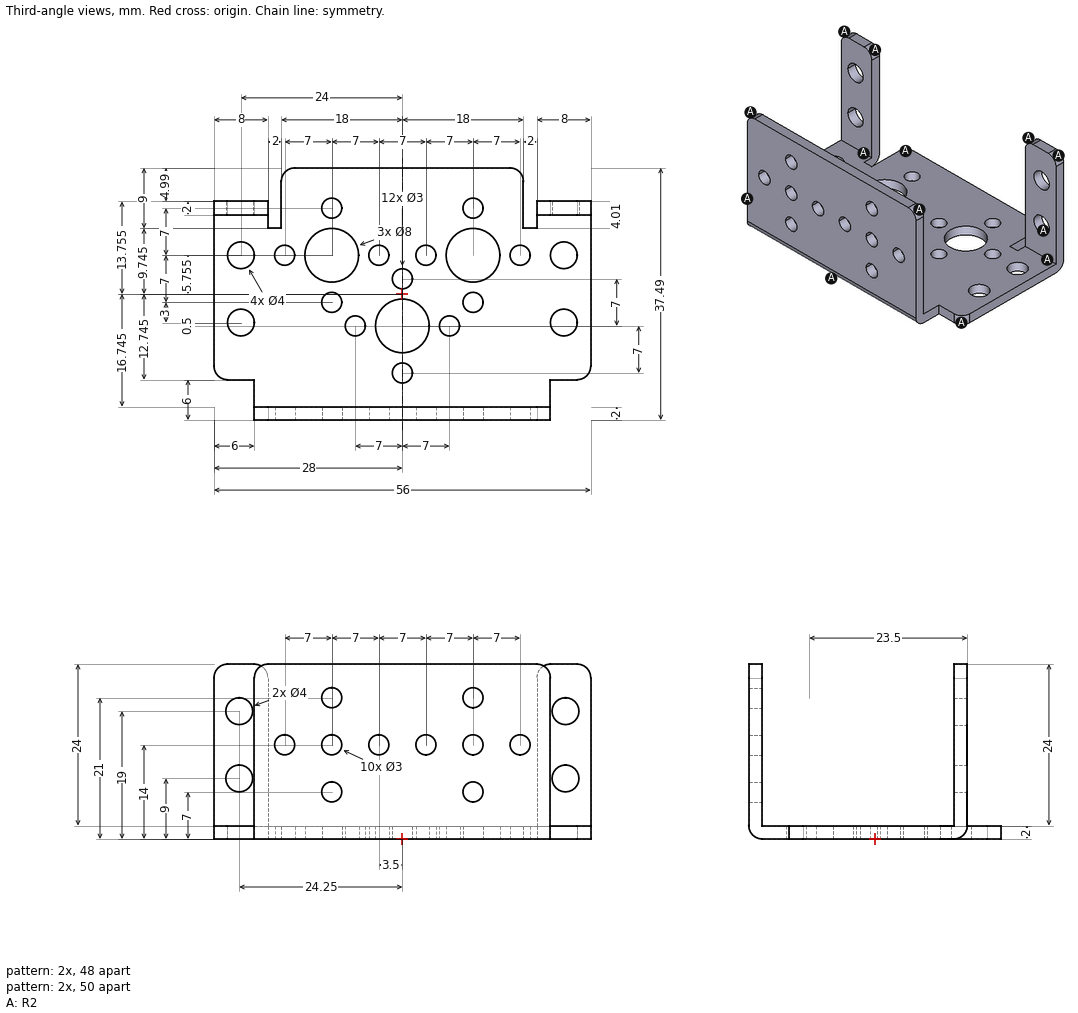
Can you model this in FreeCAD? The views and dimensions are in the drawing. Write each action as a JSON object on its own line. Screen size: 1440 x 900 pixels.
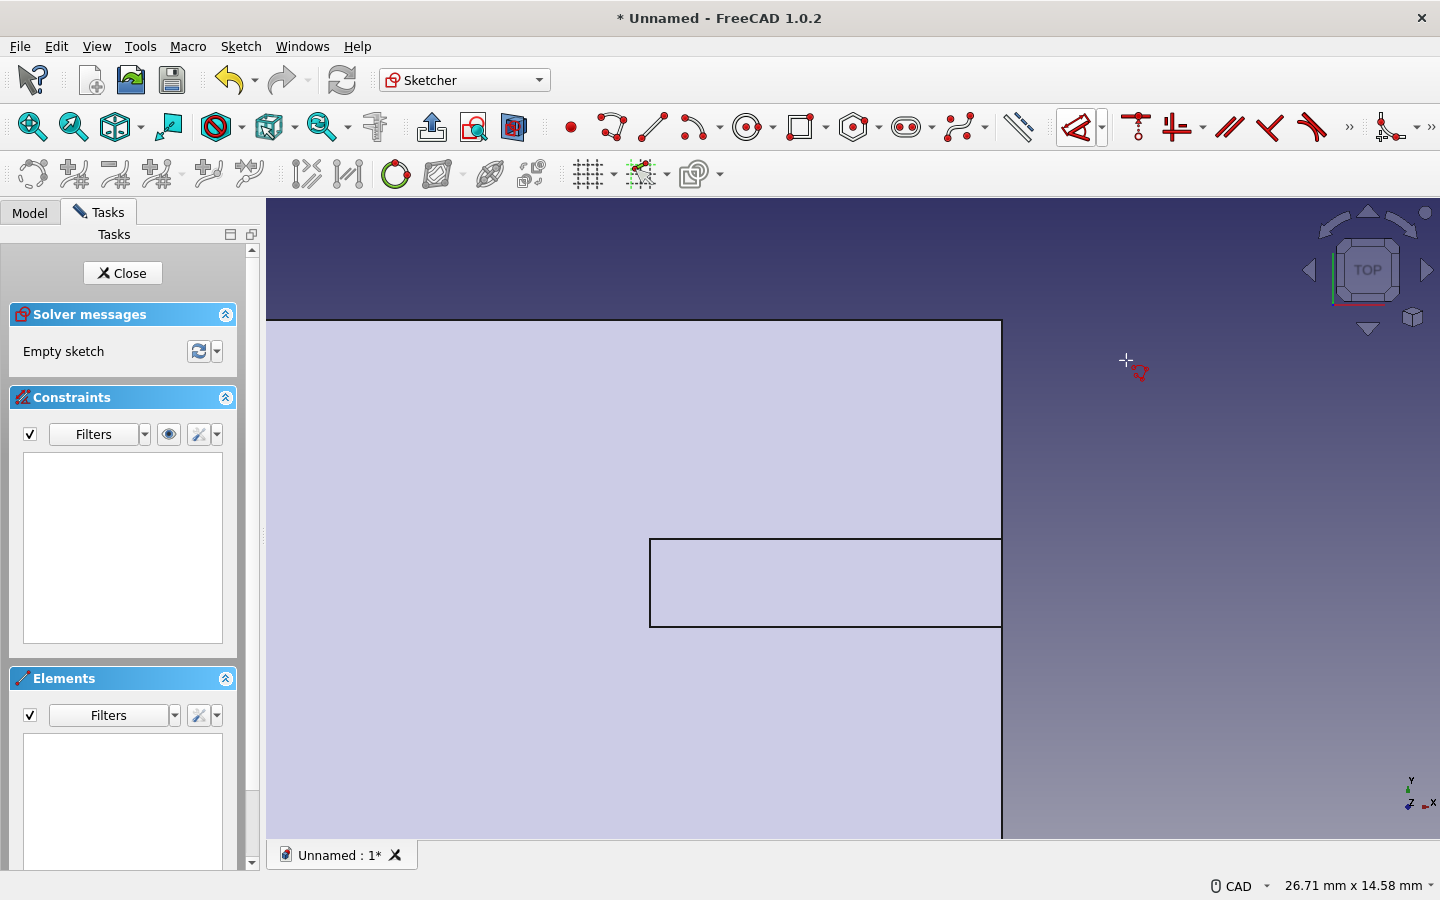
{"action": "left_click", "coordinate": [562, 716]}
{"action": "left_click", "coordinate": [650, 716]}
{"action": "left_click", "coordinate": [650, 539]}
{"action": "left_click", "coordinate": [1002, 539]}
{"action": "left_click", "coordinate": [1002, 320]}
{"action": "left_click", "coordinate": [562, 320]}
{"action": "left_click", "coordinate": [562, 717]}
{"action": "key", "text": "Escape"}
{"action": "key", "text": "Escape"}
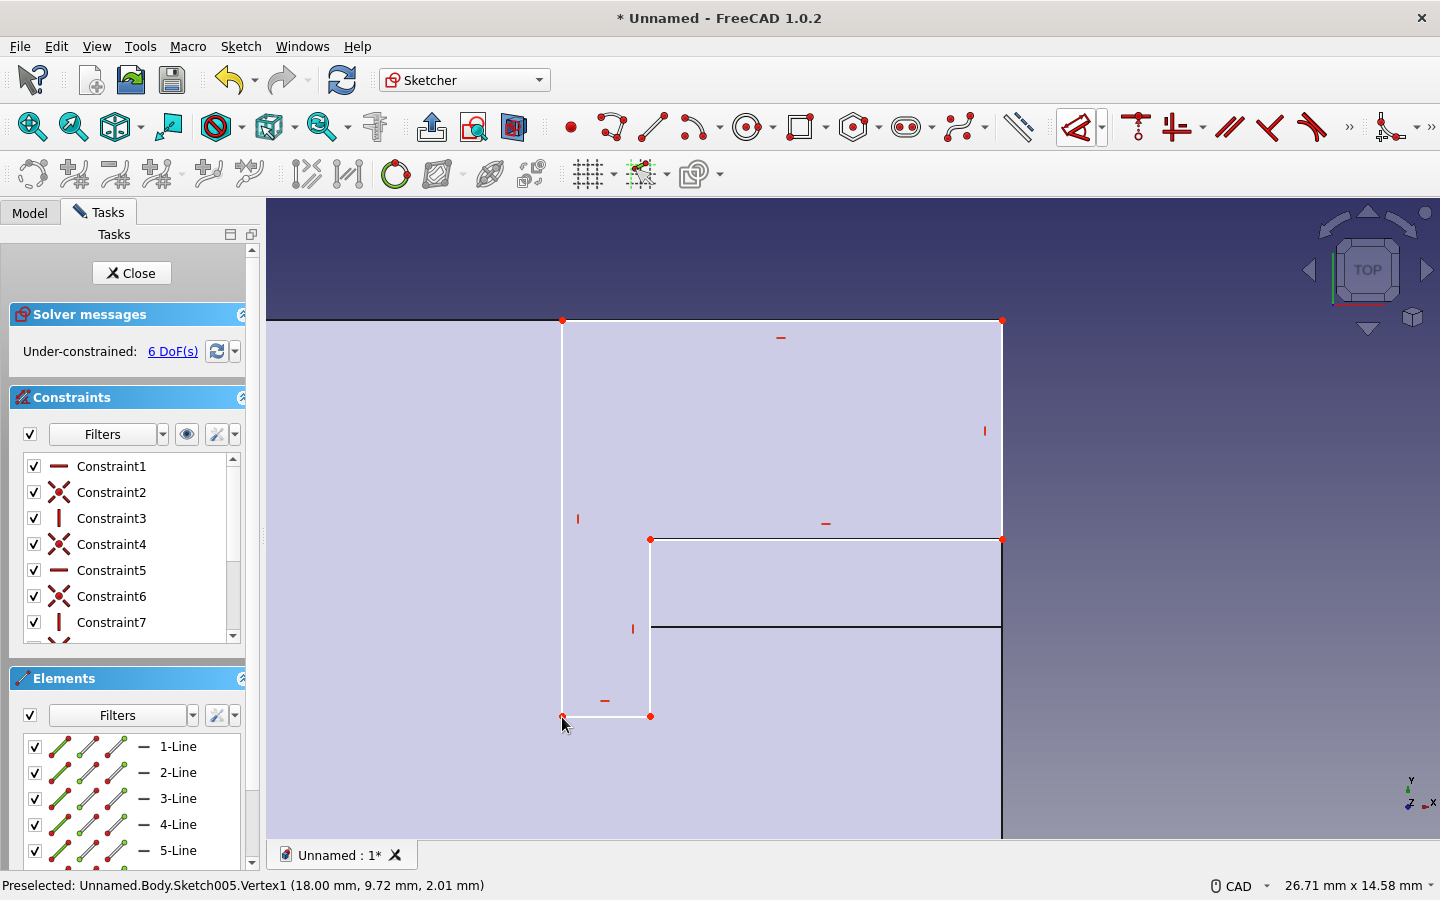
{"action": "left_click", "coordinate": [588, 717]}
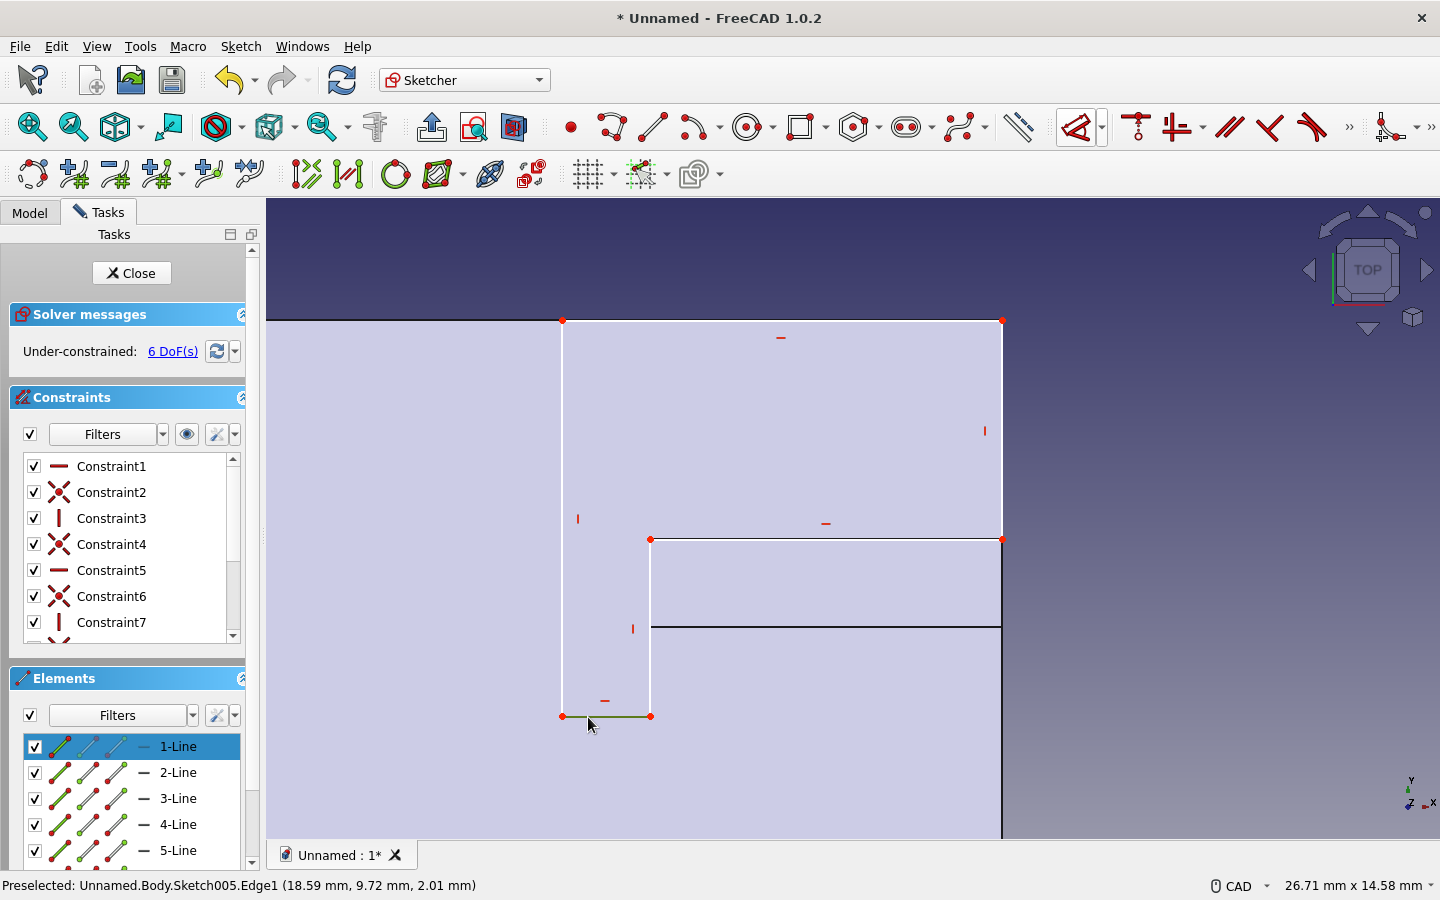
{"action": "key", "text": "l"}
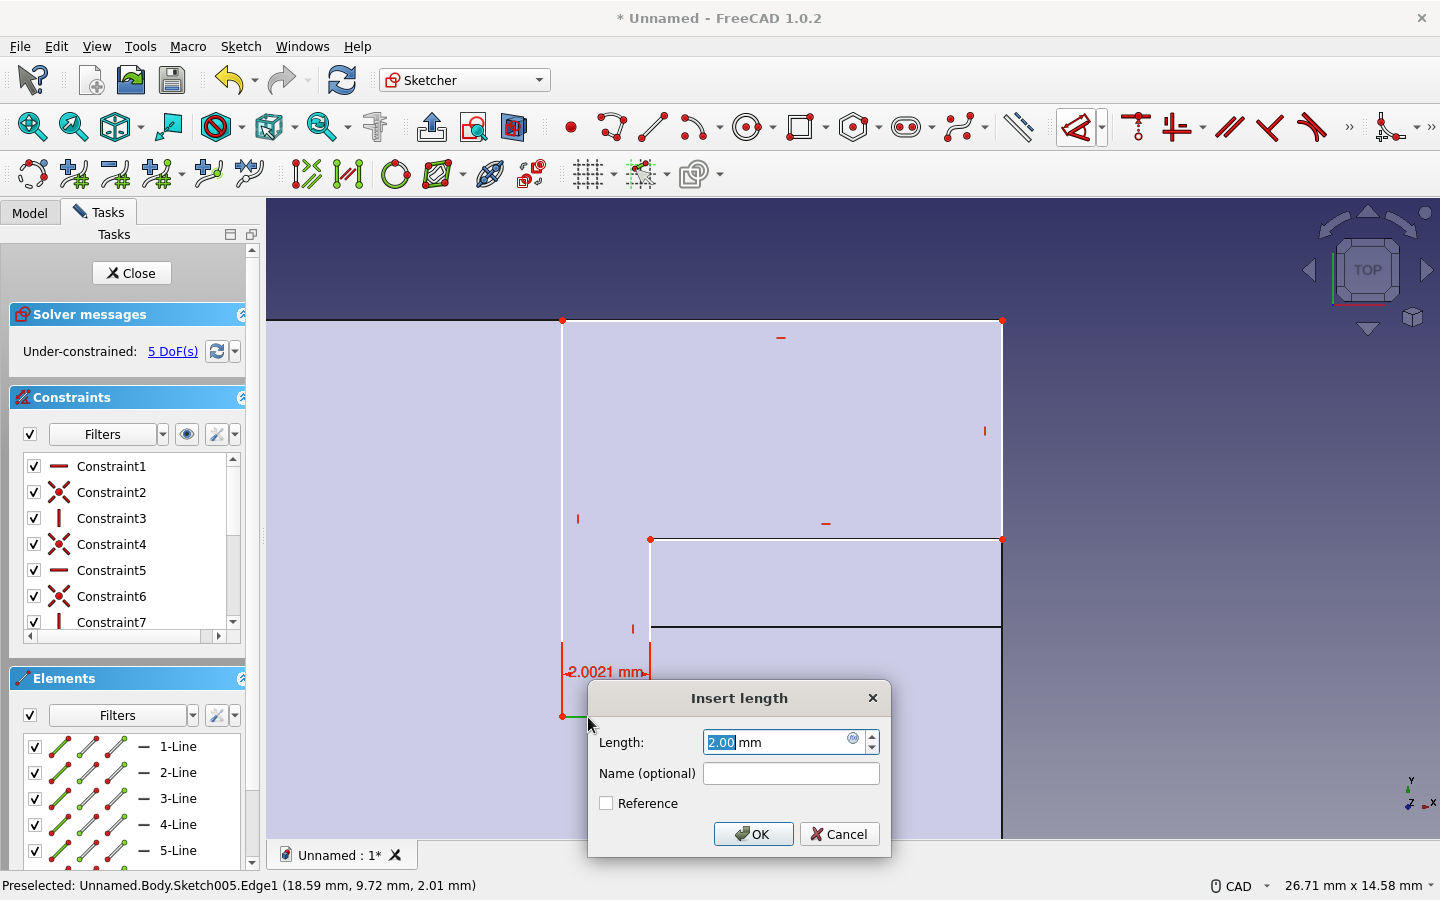
{"action": "type", "text": "2"}
{"action": "key", "text": "Return"}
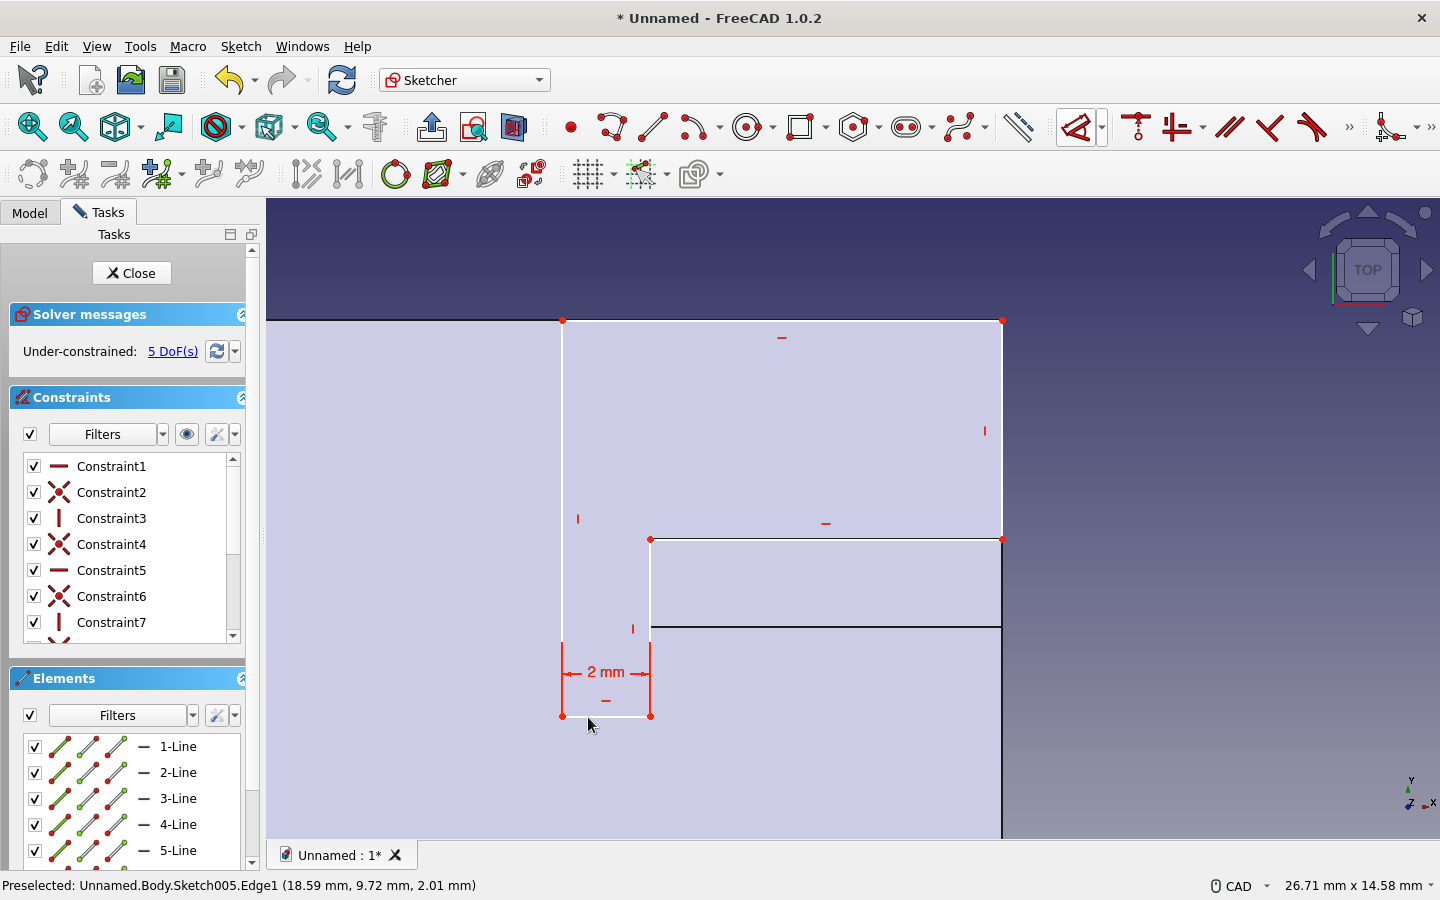
{"action": "left_click", "coordinate": [756, 540]}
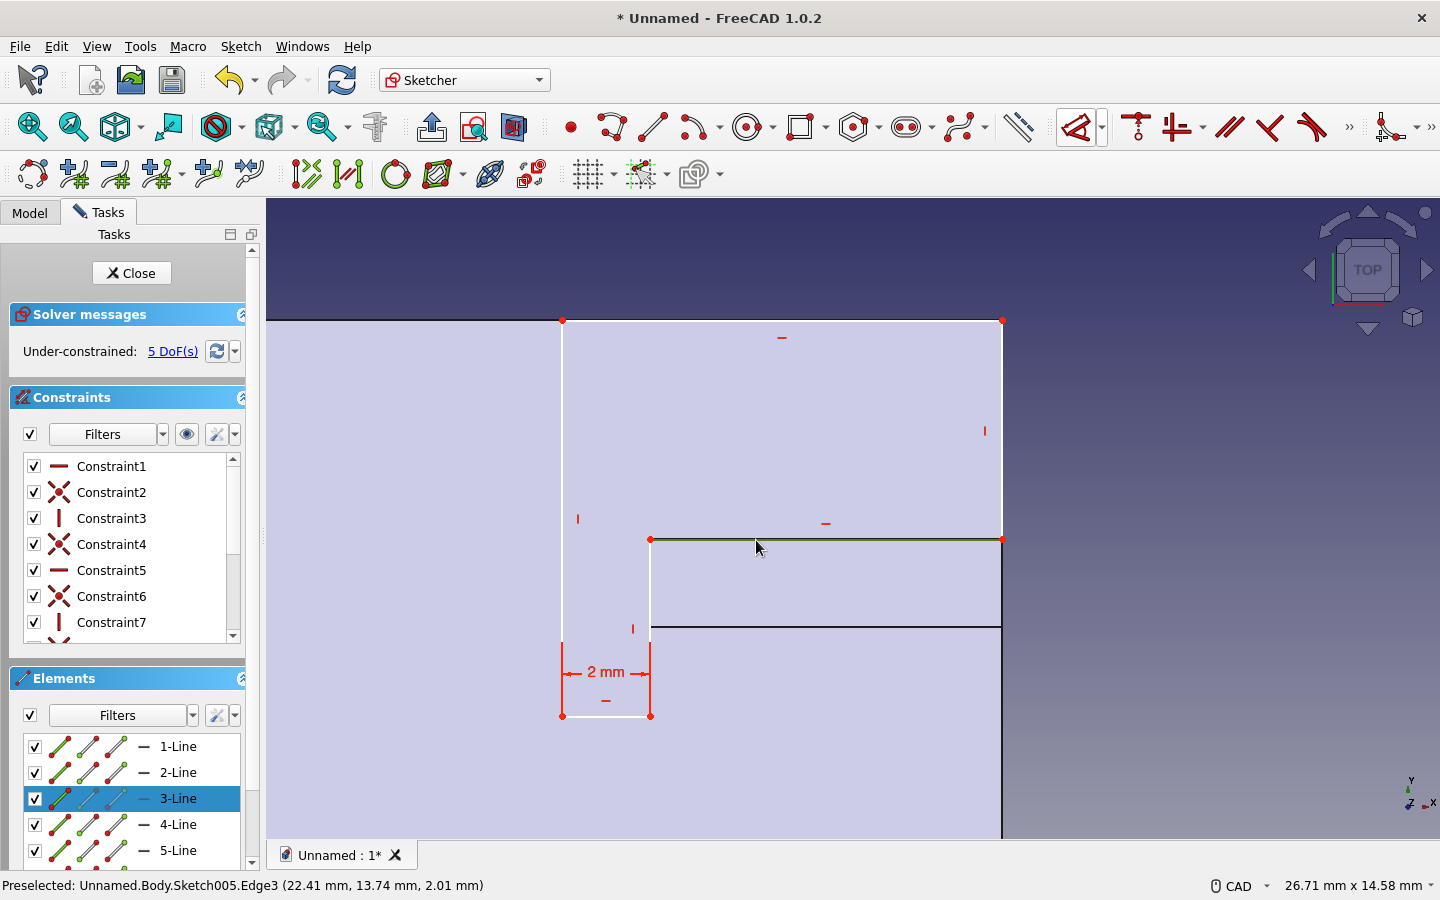
{"action": "key", "text": "l"}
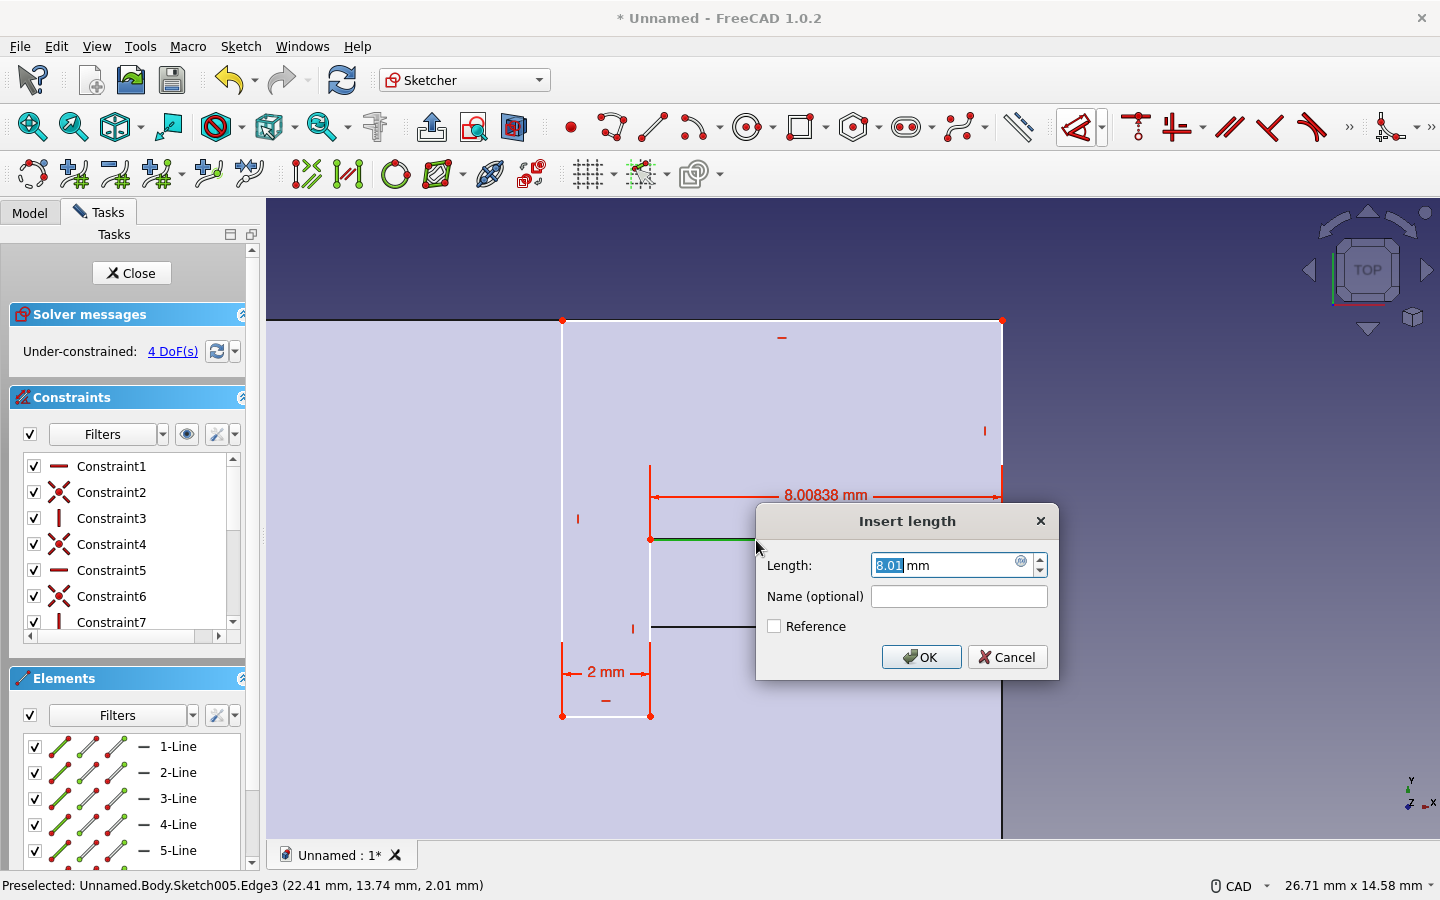
{"action": "type", "text": "8"}
{"action": "key", "text": "Return"}